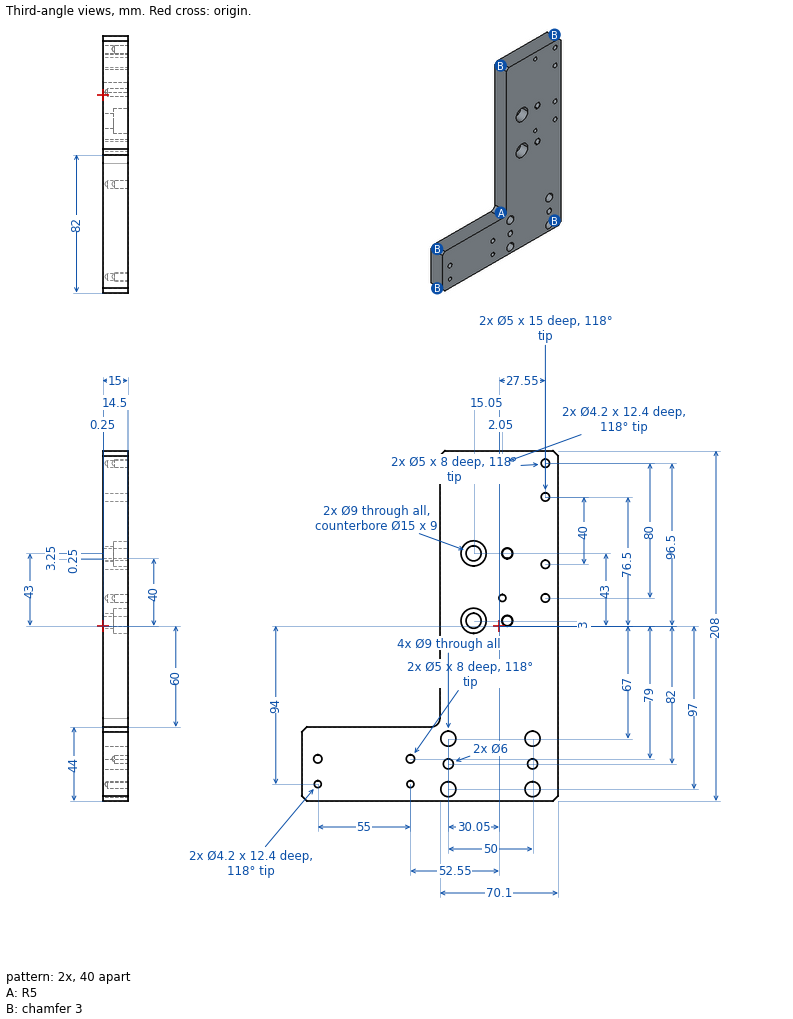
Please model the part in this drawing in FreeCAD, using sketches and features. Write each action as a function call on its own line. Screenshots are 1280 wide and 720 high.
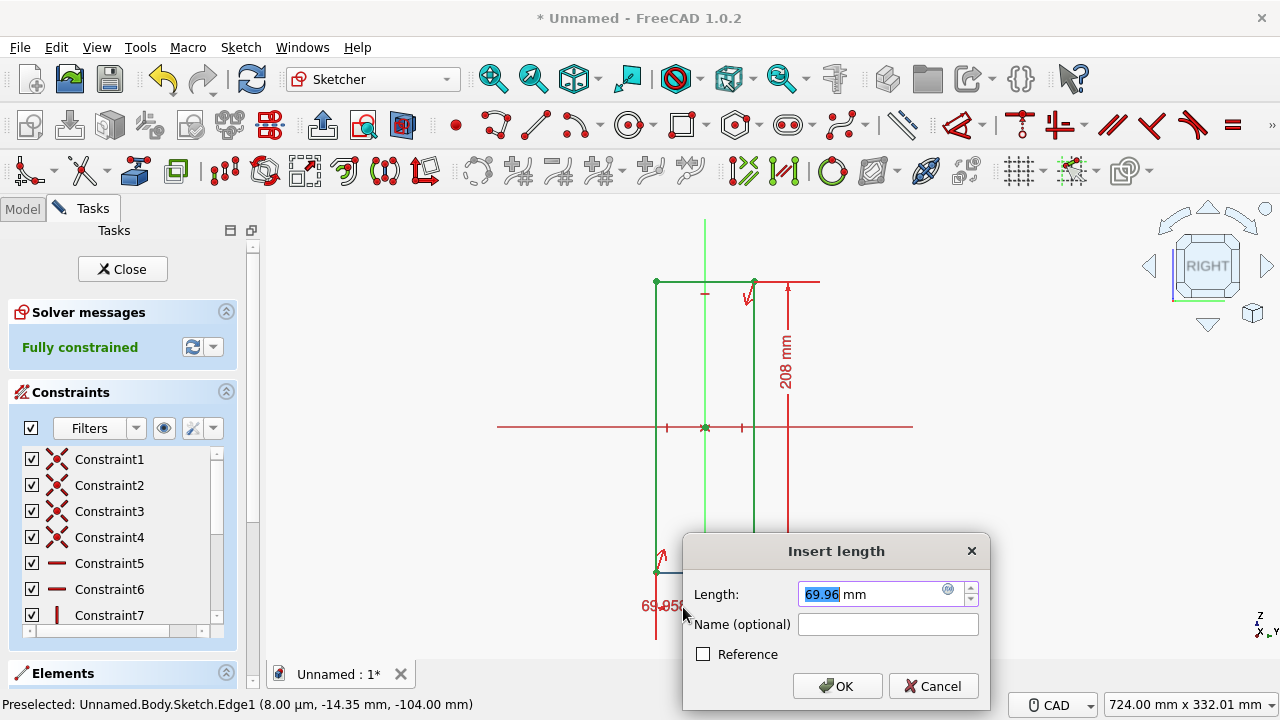
text(70.1)
key(Return)
key(Escape)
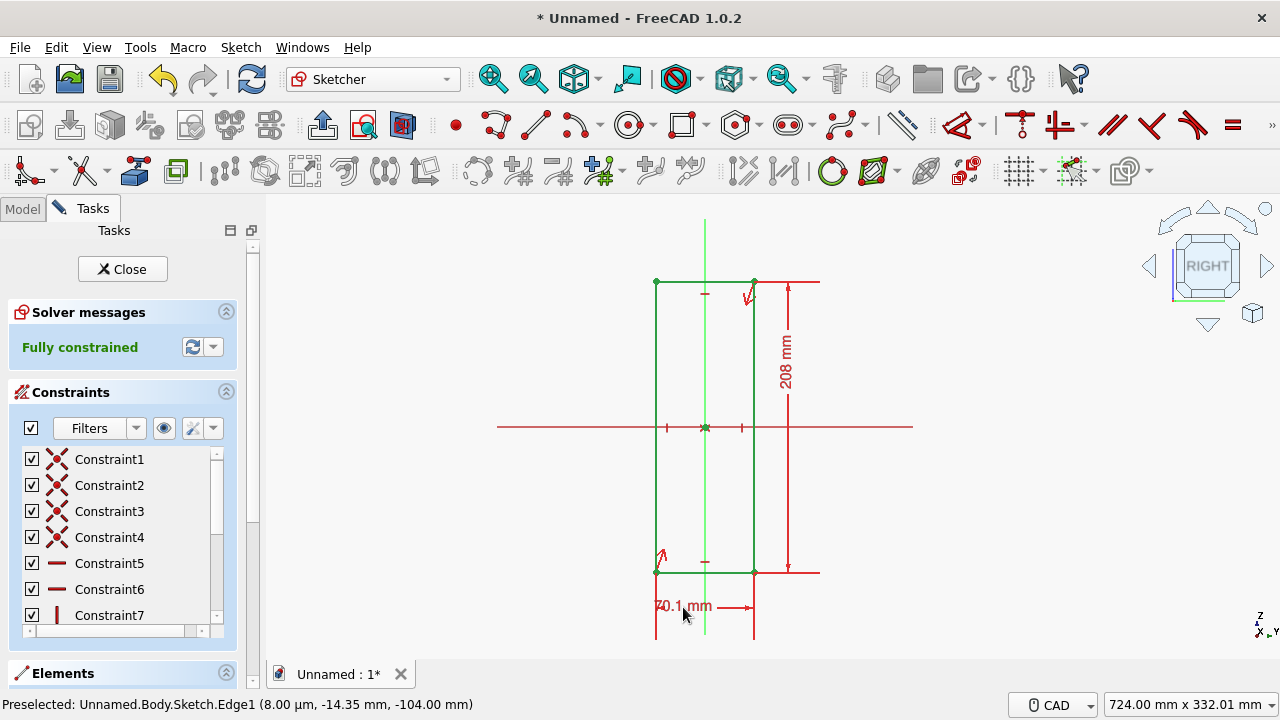
click(123, 269)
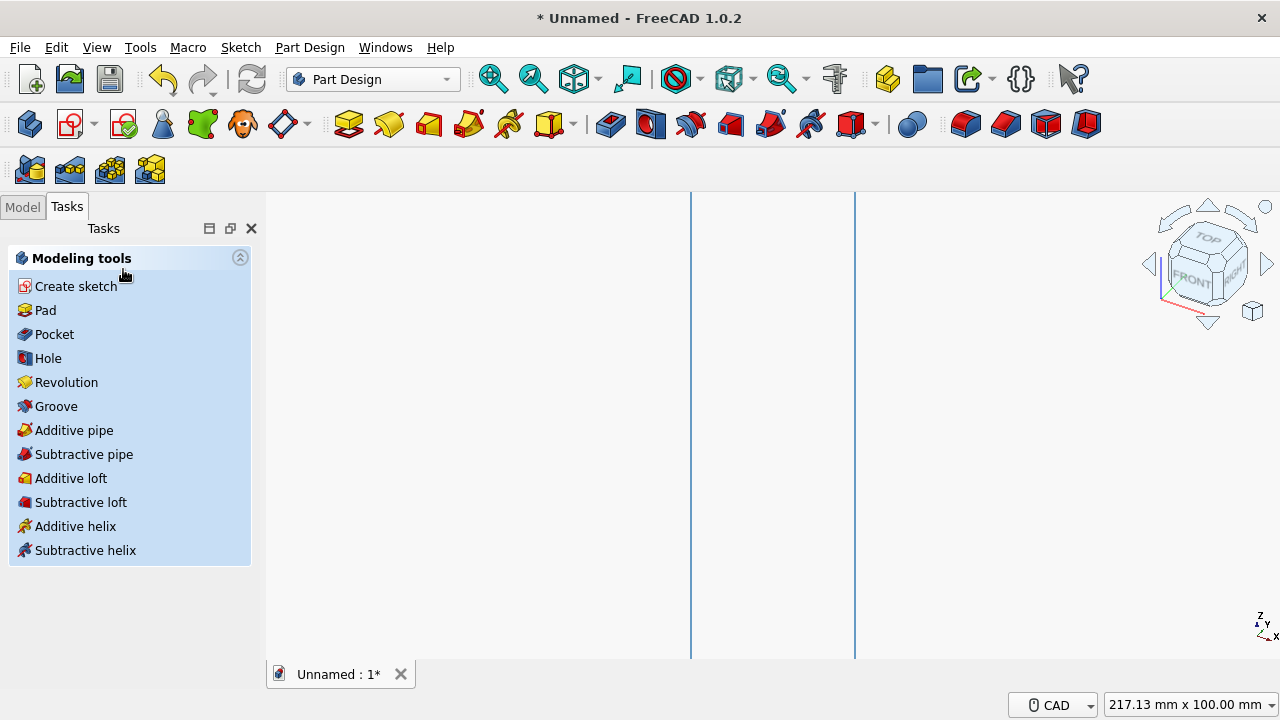
click(350, 124)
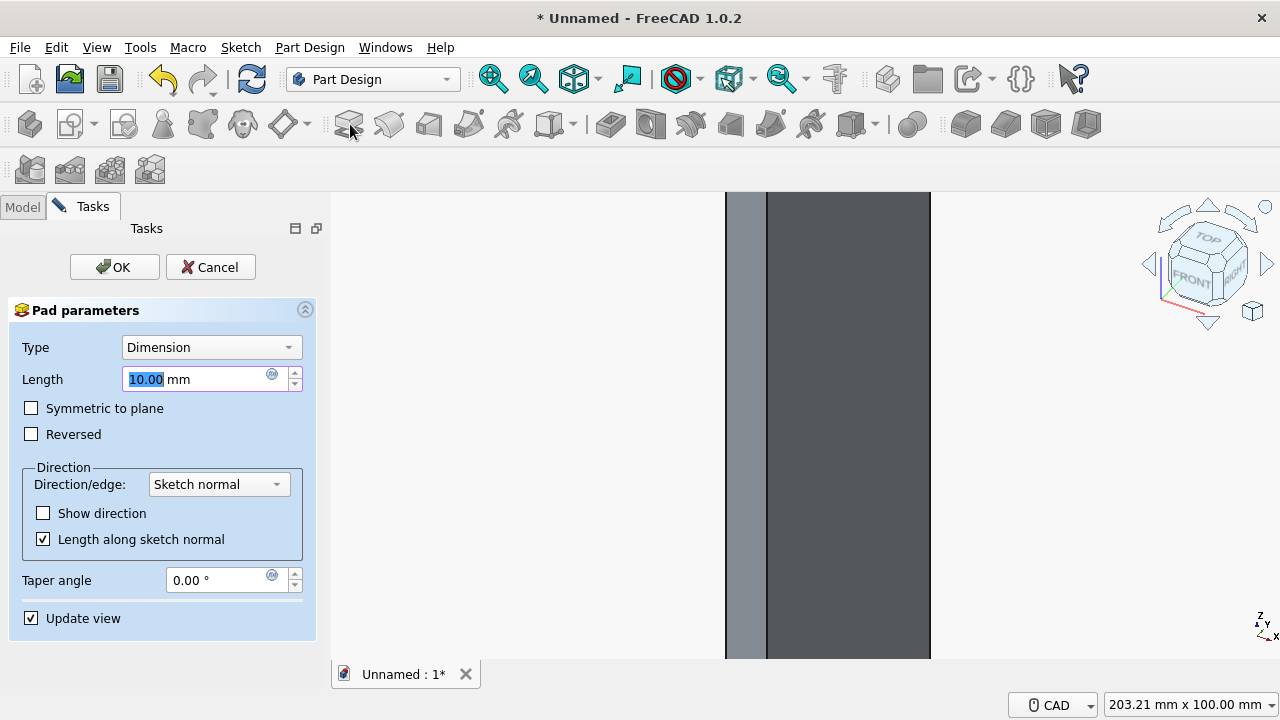
text(15)
key(Tab)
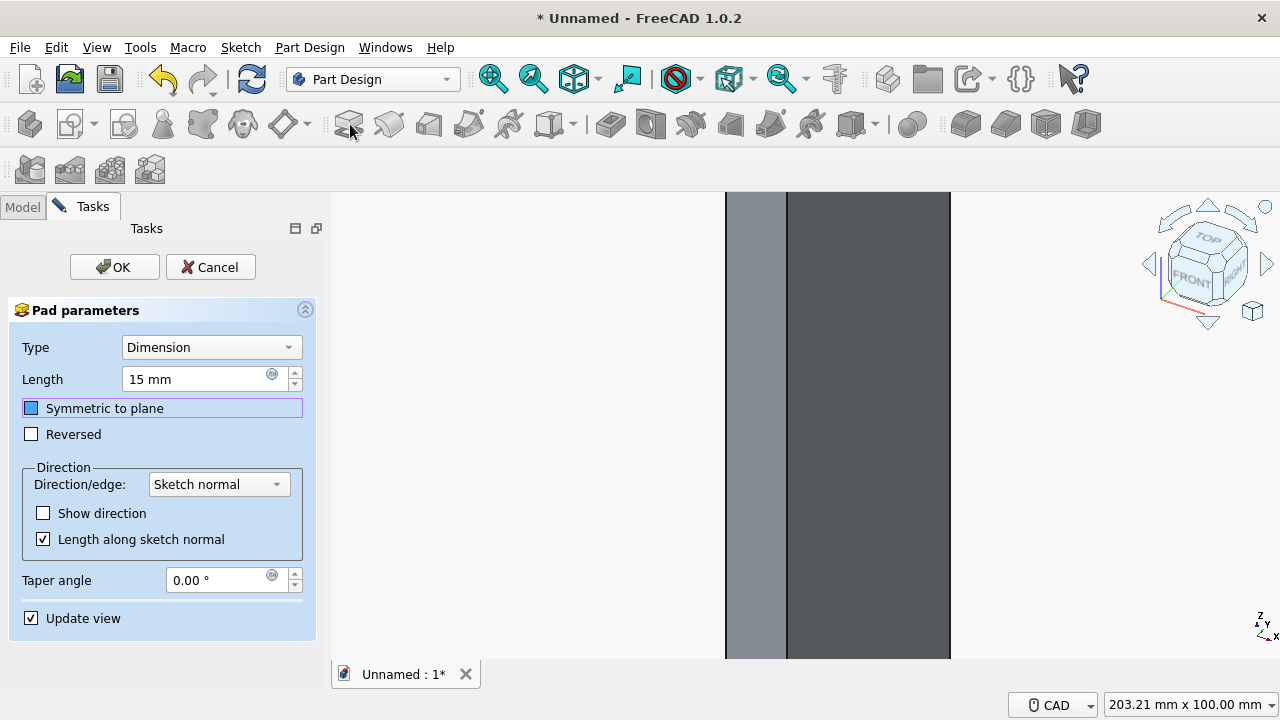
click(115, 267)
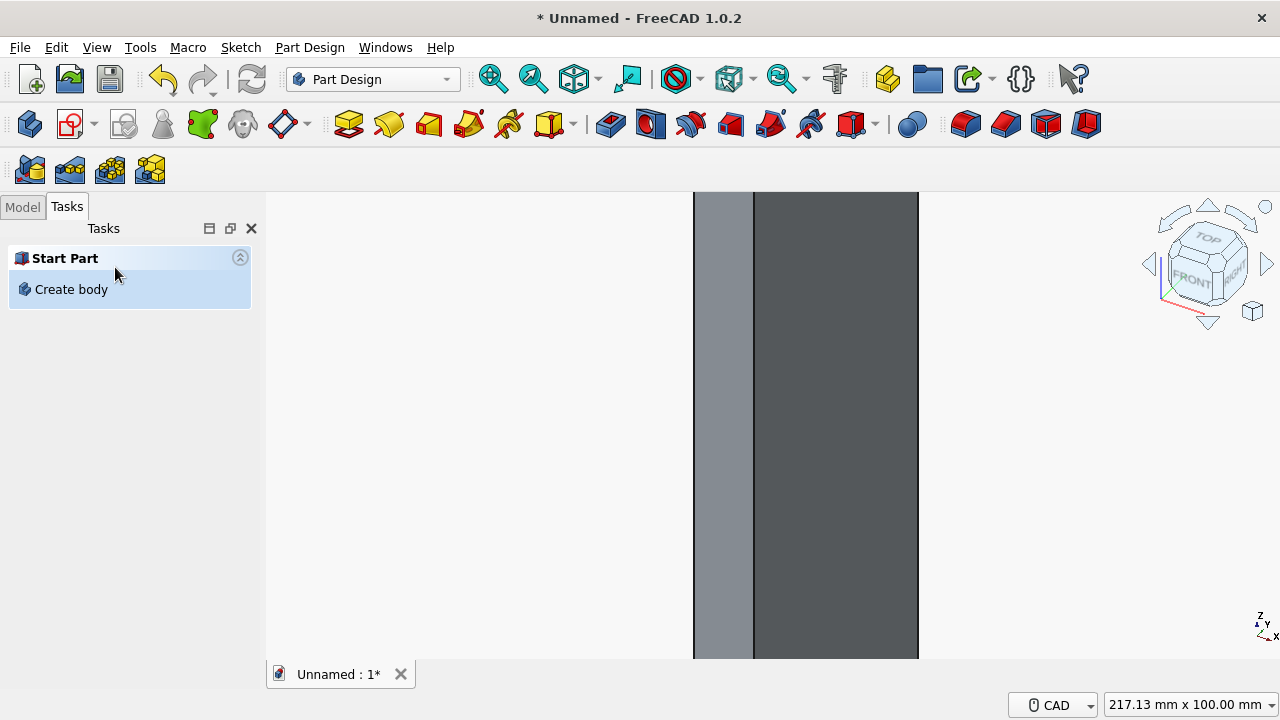
click(494, 80)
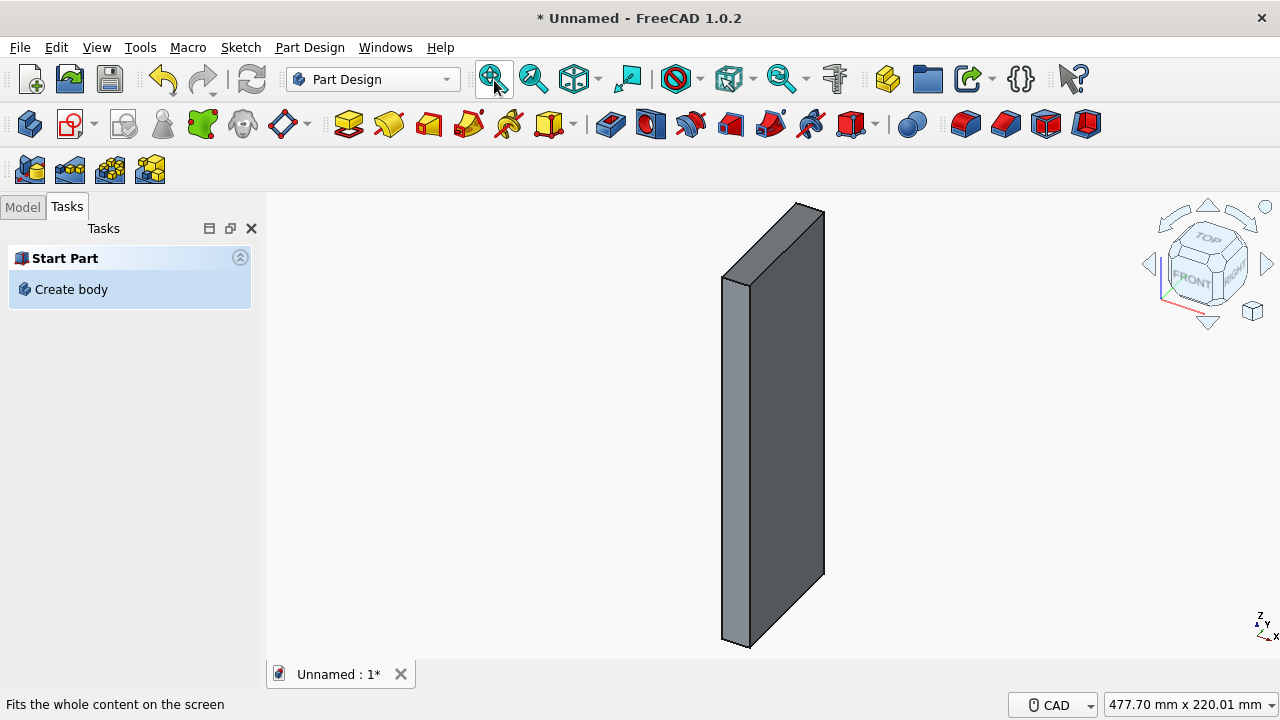
click(787, 532)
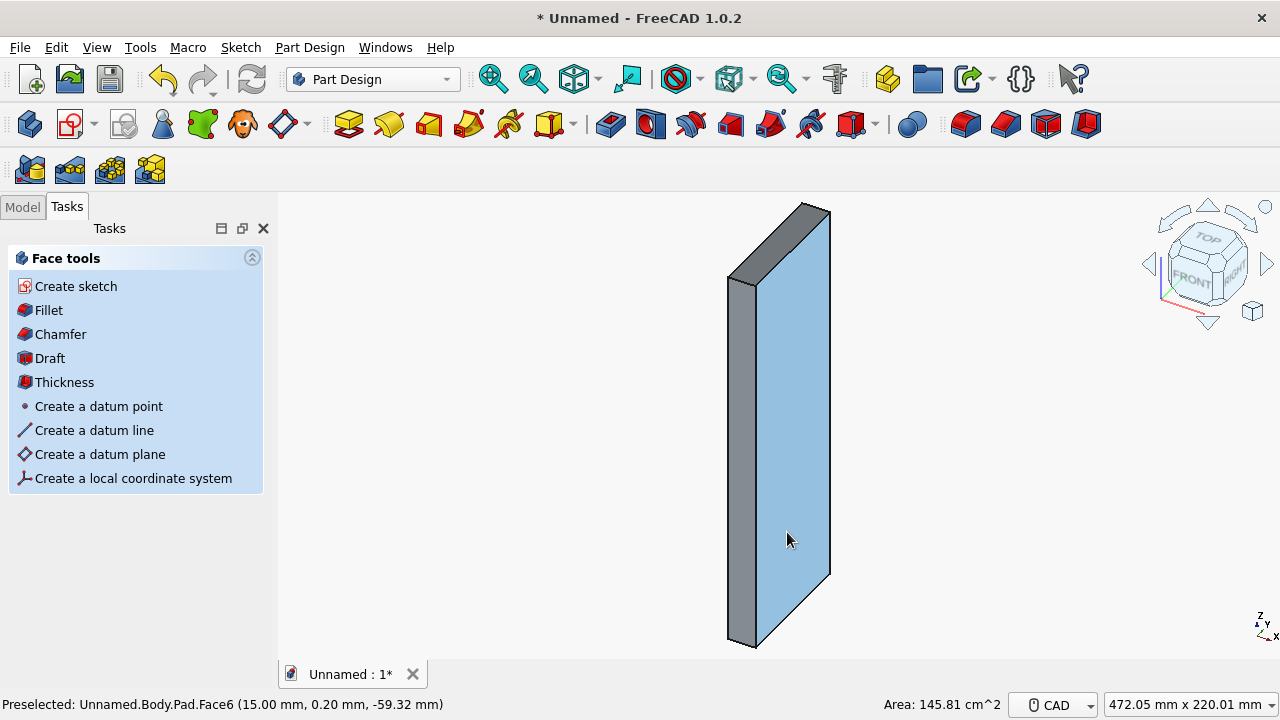
click(70, 124)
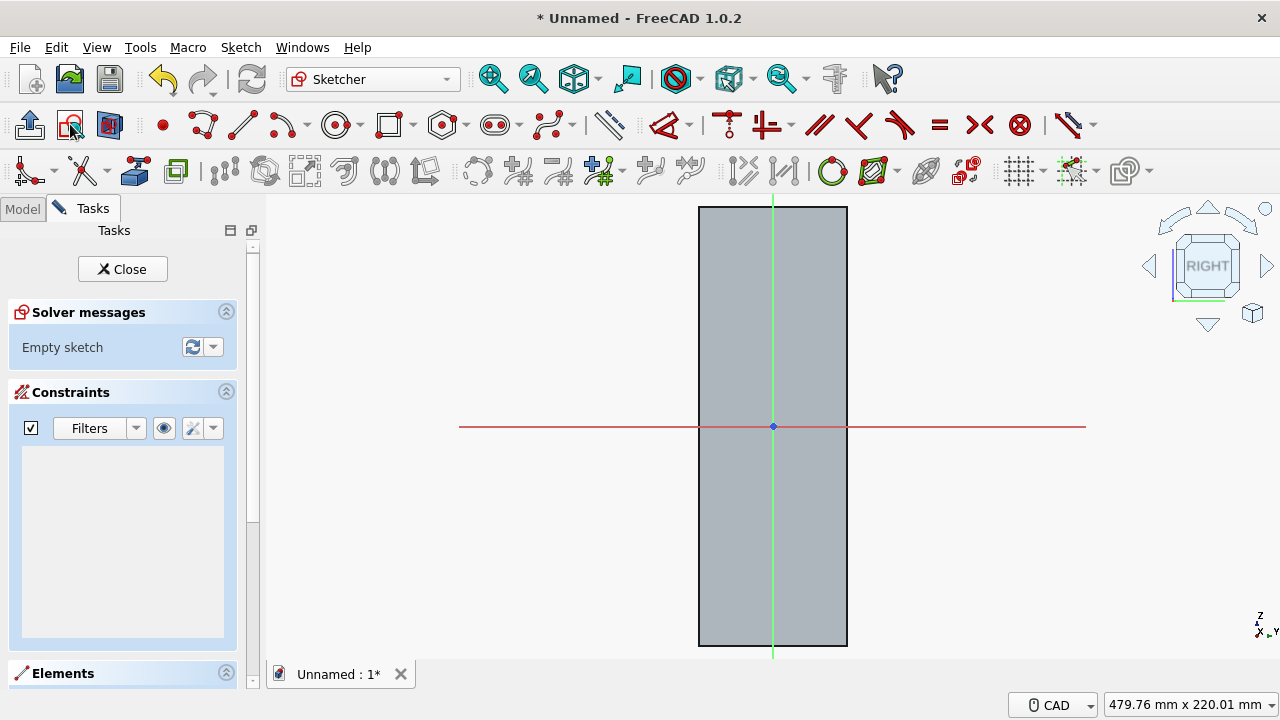
scroll(780, 350, up, 5)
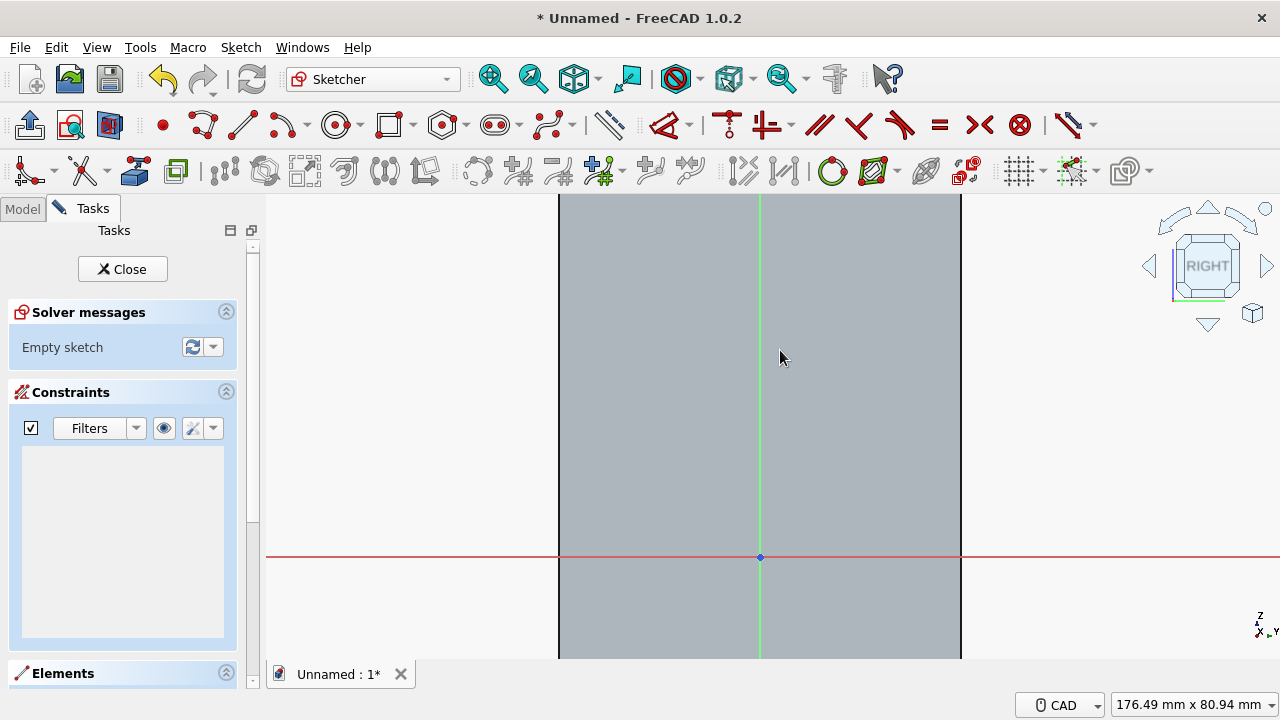
click(336, 126)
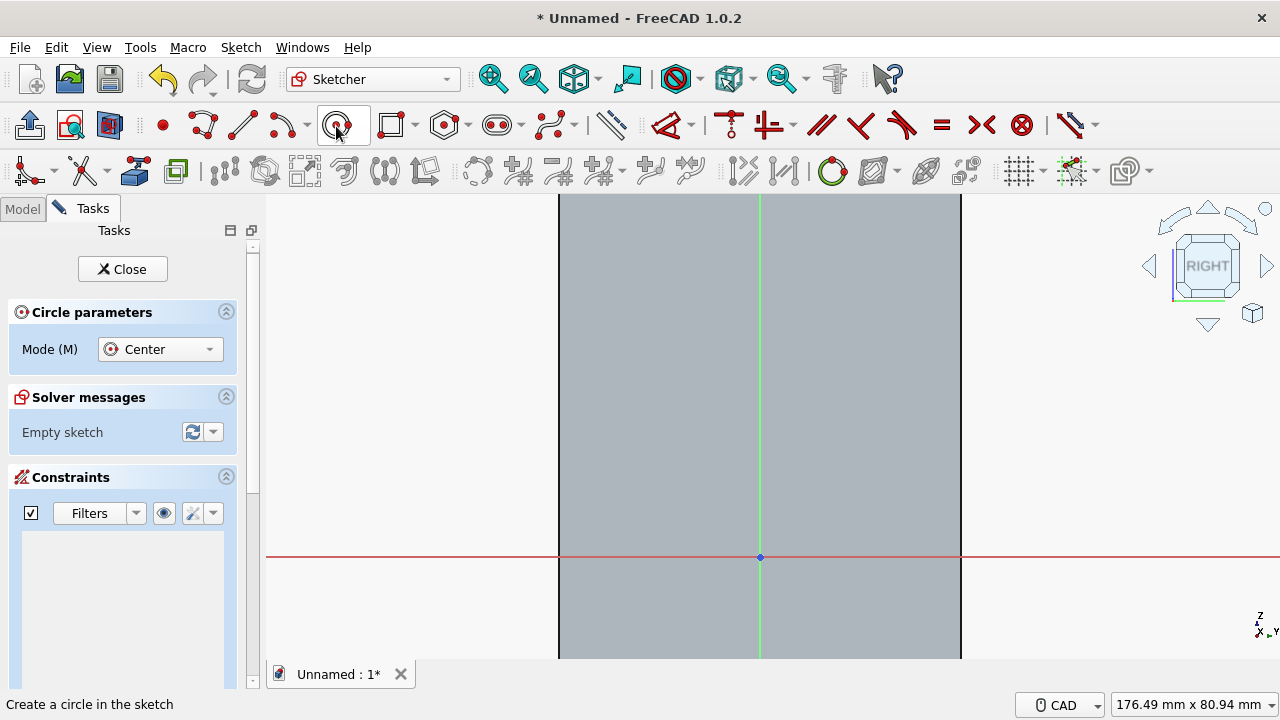
click(674, 310)
click(692, 292)